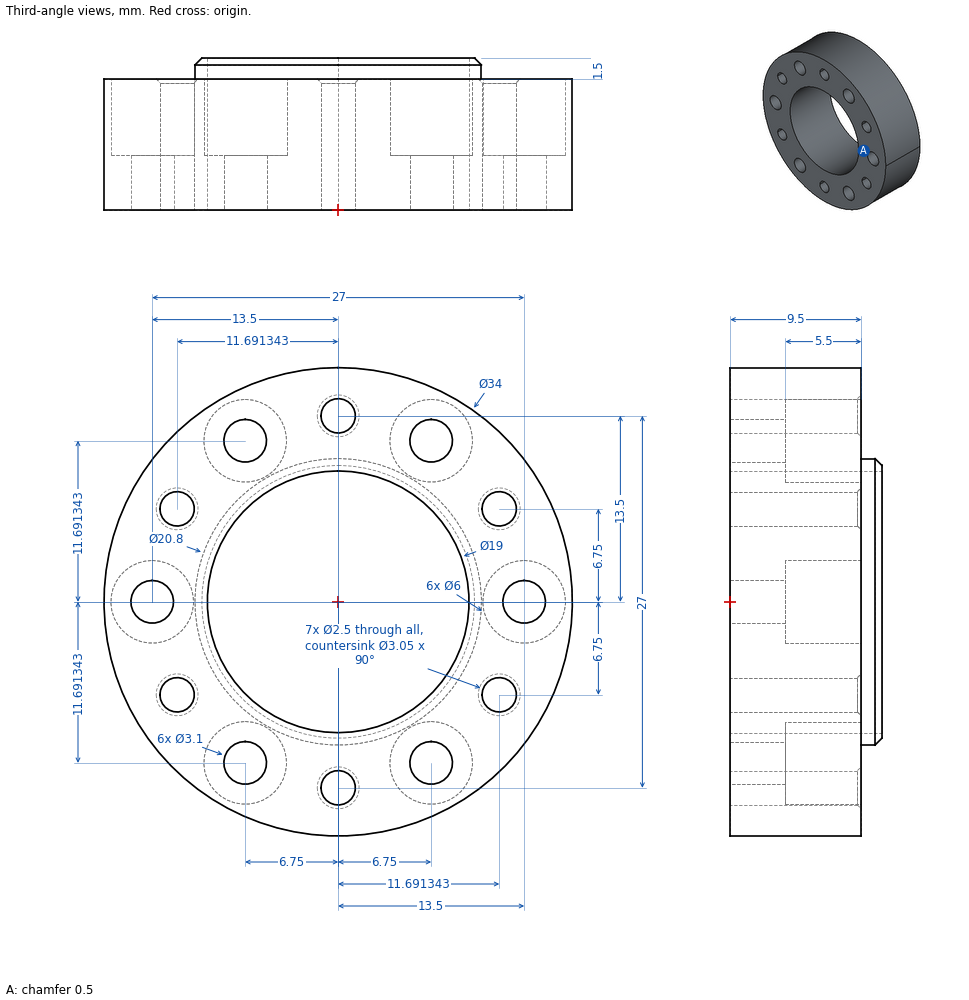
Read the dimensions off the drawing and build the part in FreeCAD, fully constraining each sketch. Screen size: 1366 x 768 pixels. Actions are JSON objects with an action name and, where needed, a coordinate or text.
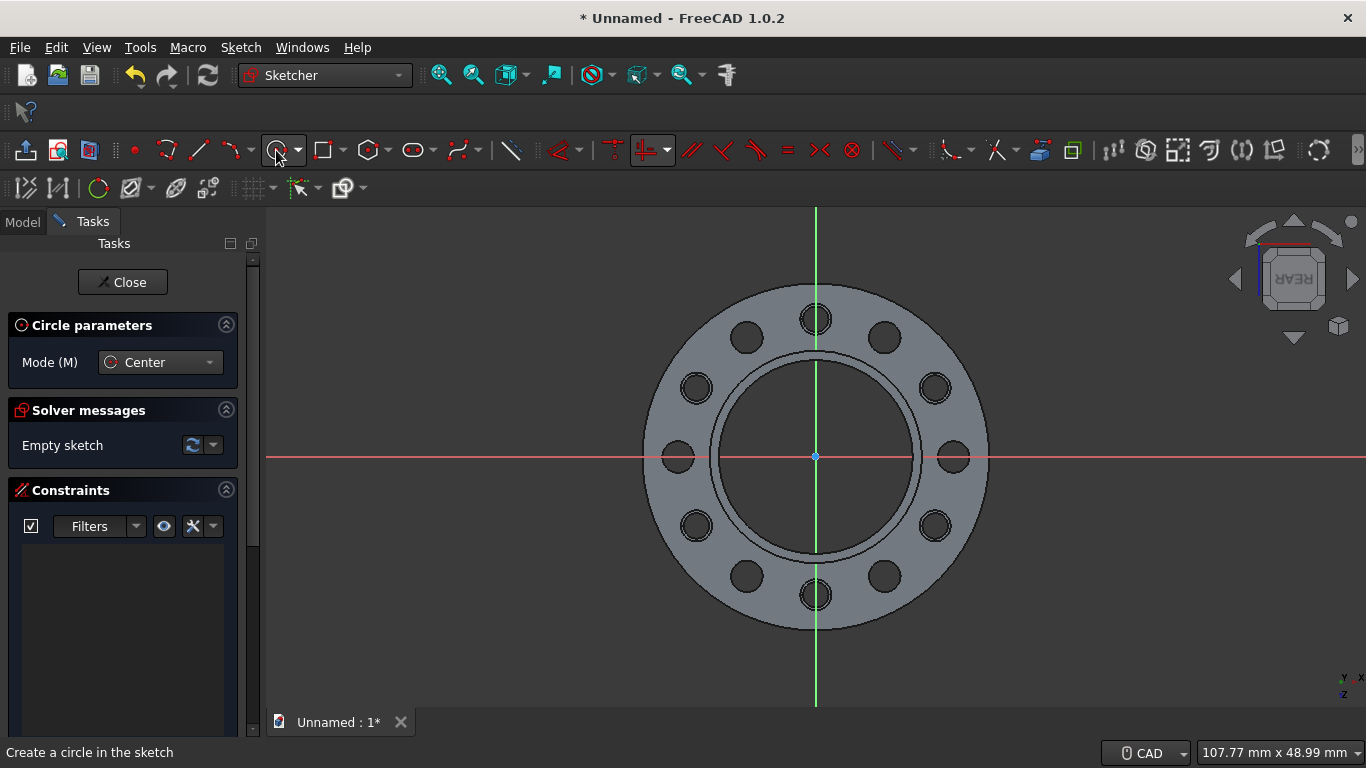
{"action": "left_click", "coordinate": [954, 457]}
{"action": "mouse_move", "coordinate": [975, 435]}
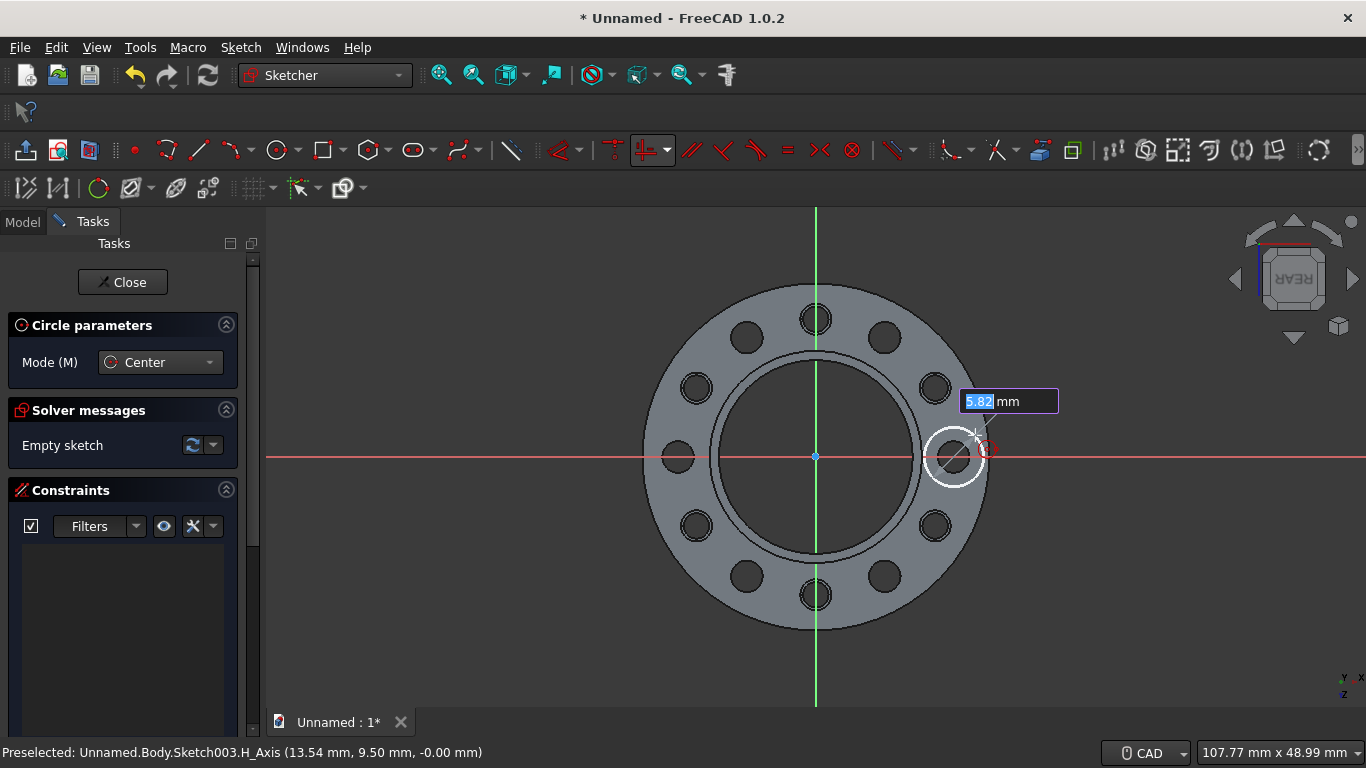
{"action": "type", "text": "6"}
{"action": "key", "text": "Return"}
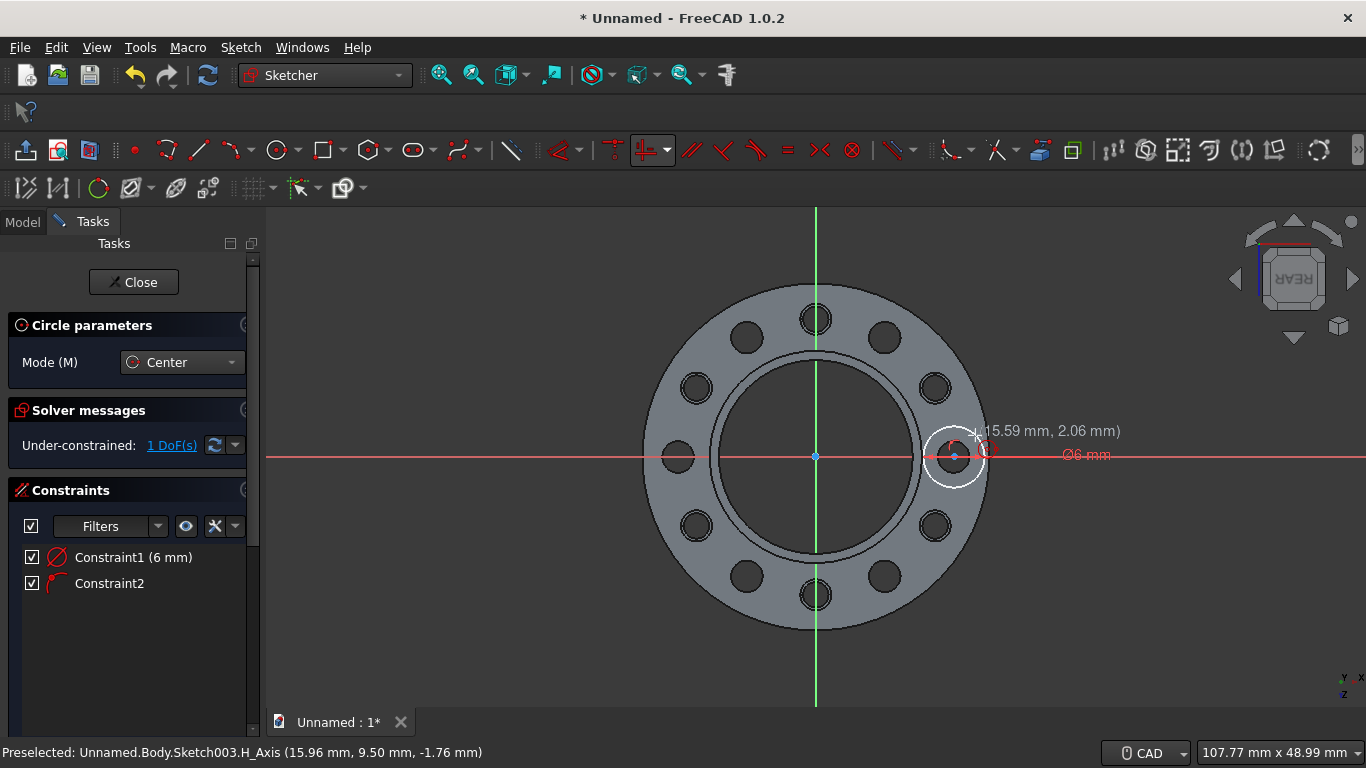
{"action": "left_click", "coordinate": [885, 576]}
{"action": "mouse_move", "coordinate": [906, 555]}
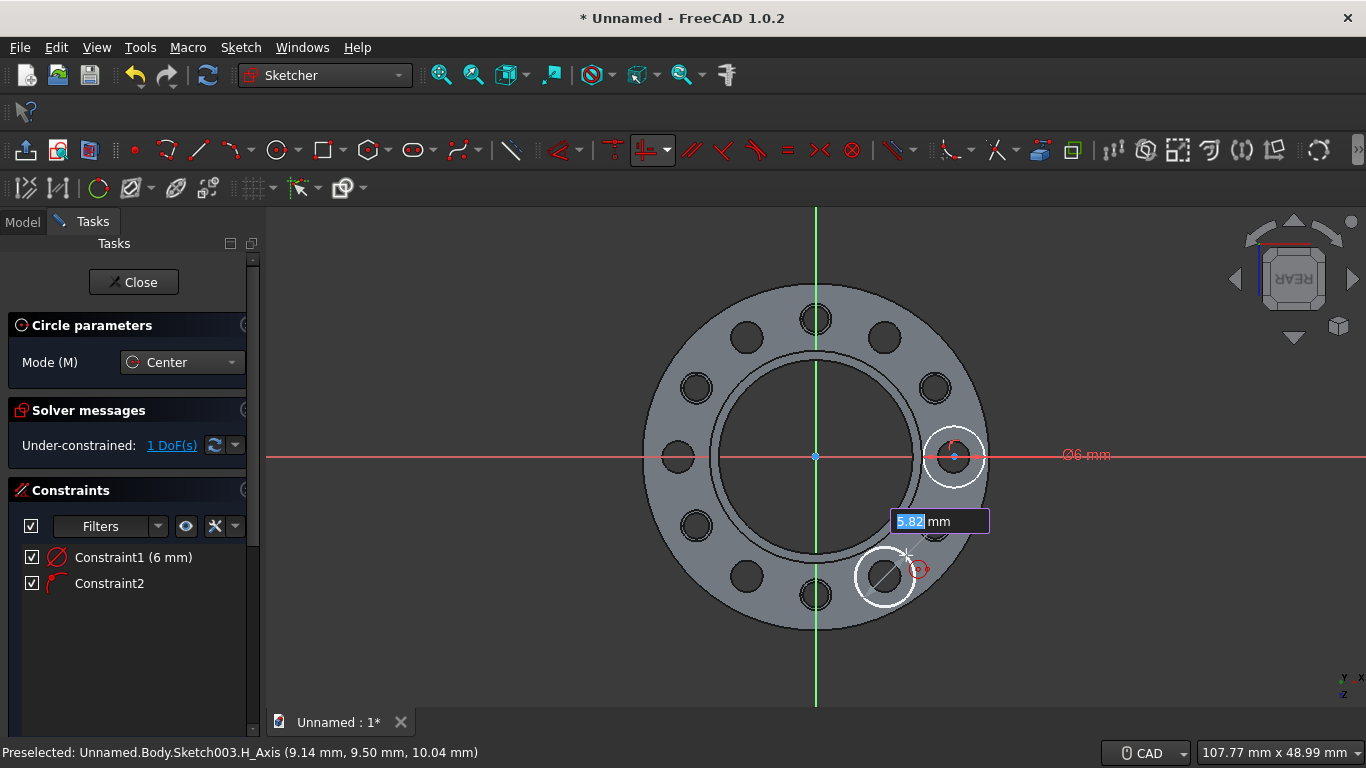
{"action": "type", "text": "6"}
{"action": "key", "text": "Return"}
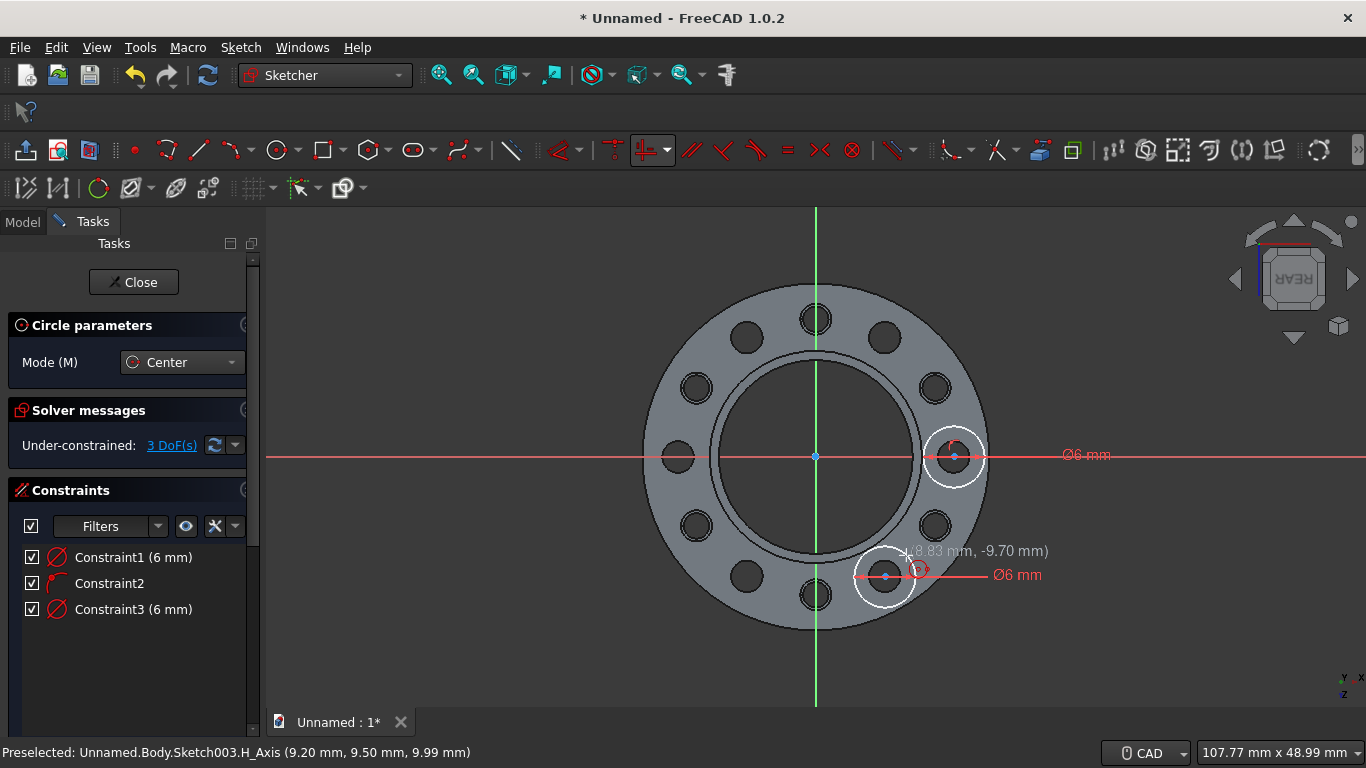
{"action": "left_click", "coordinate": [747, 576]}
{"action": "mouse_move", "coordinate": [769, 555]}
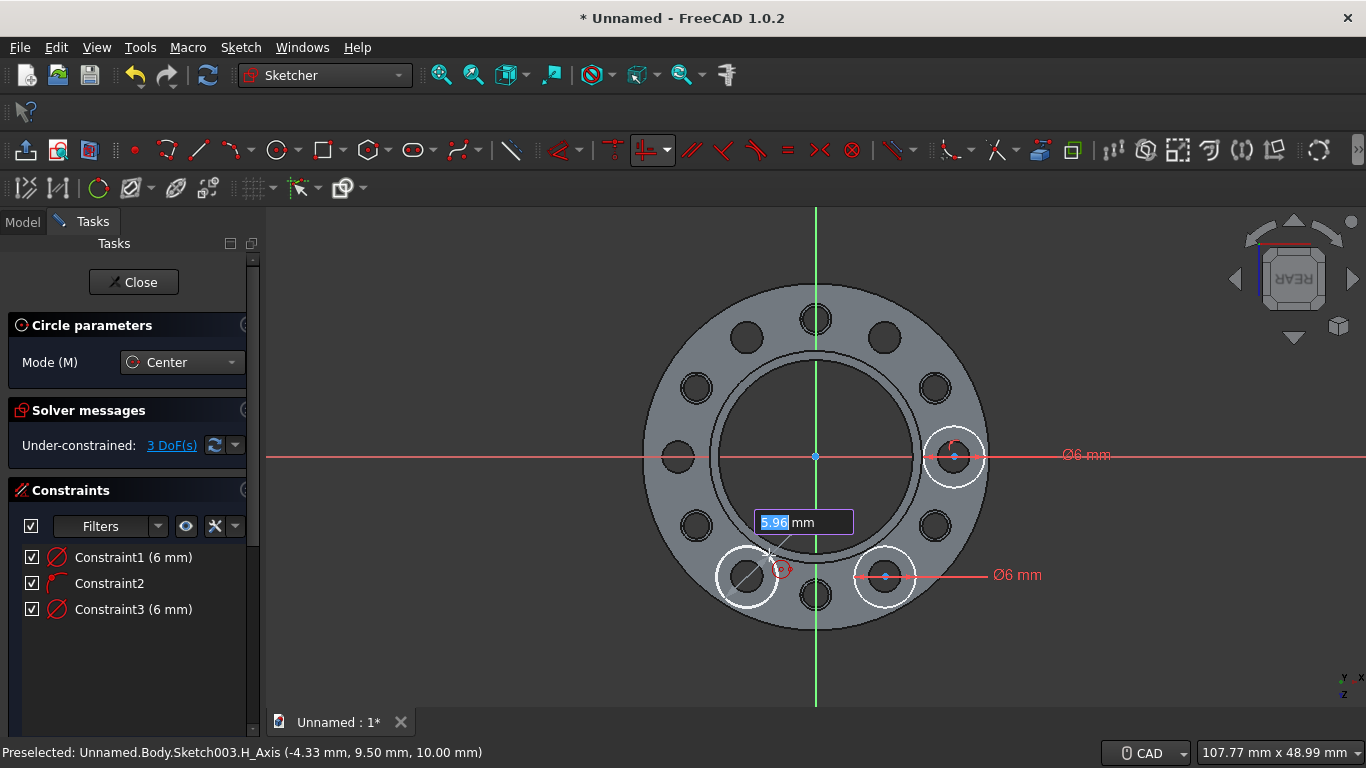
{"action": "type", "text": "6"}
{"action": "key", "text": "Return"}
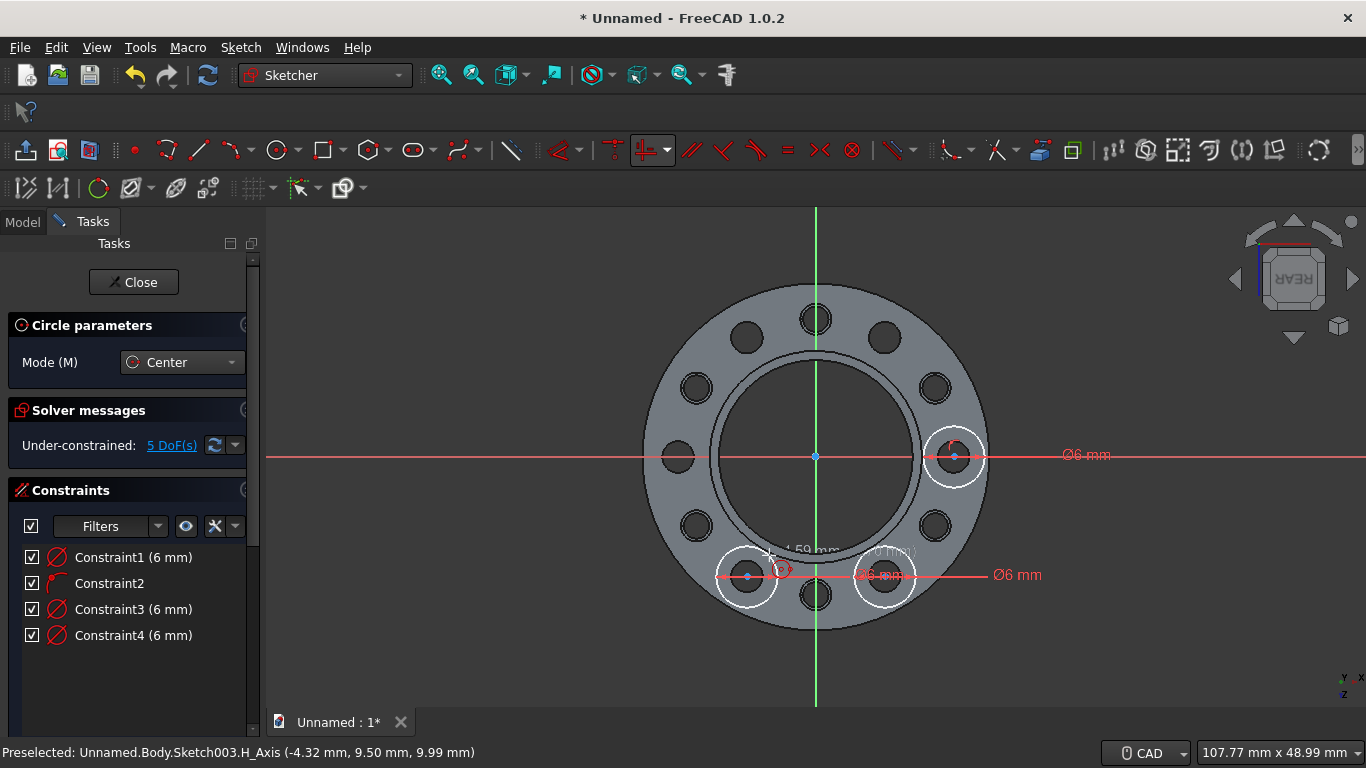
{"action": "left_click", "coordinate": [678, 457]}
{"action": "mouse_move", "coordinate": [700, 435]}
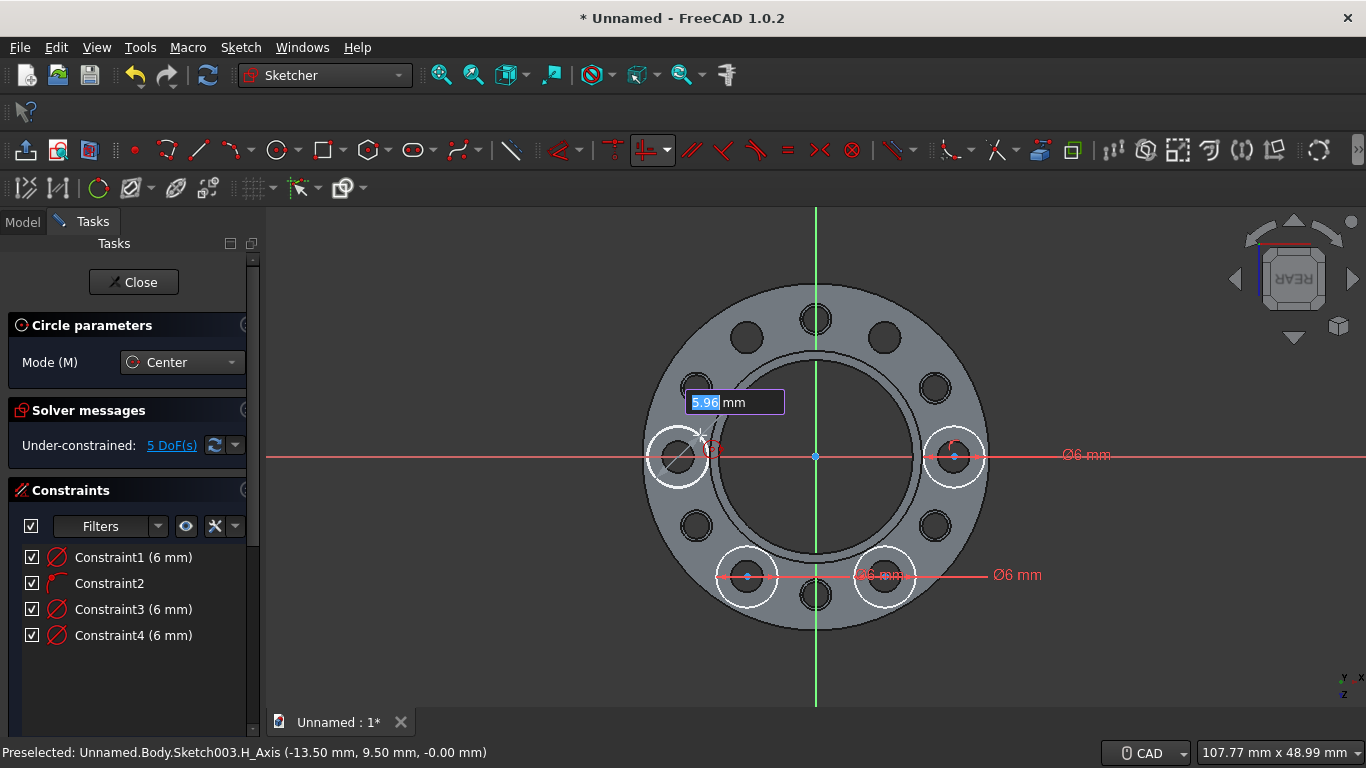
{"action": "type", "text": "6"}
{"action": "key", "text": "Return"}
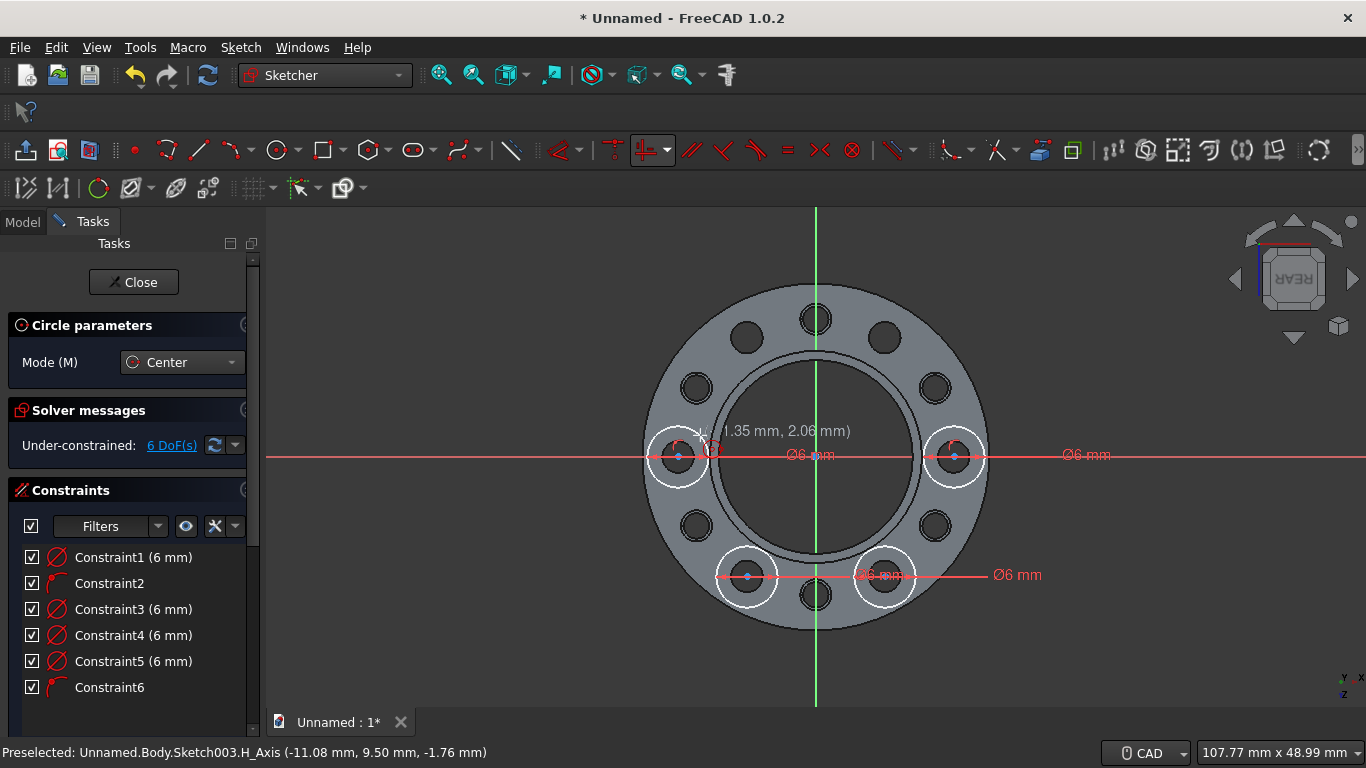
{"action": "left_click", "coordinate": [747, 338]}
{"action": "mouse_move", "coordinate": [769, 316]}